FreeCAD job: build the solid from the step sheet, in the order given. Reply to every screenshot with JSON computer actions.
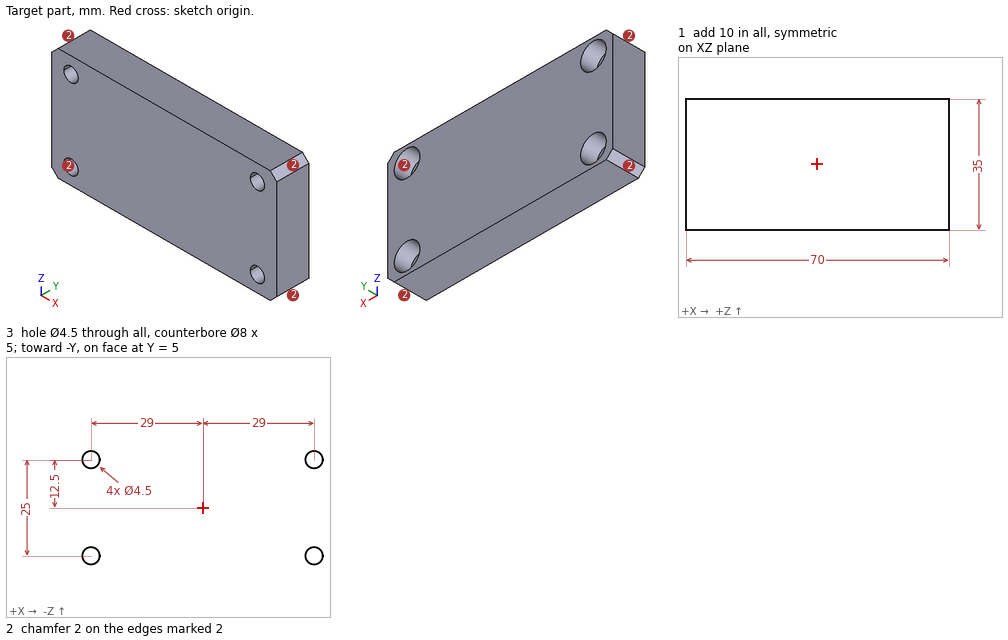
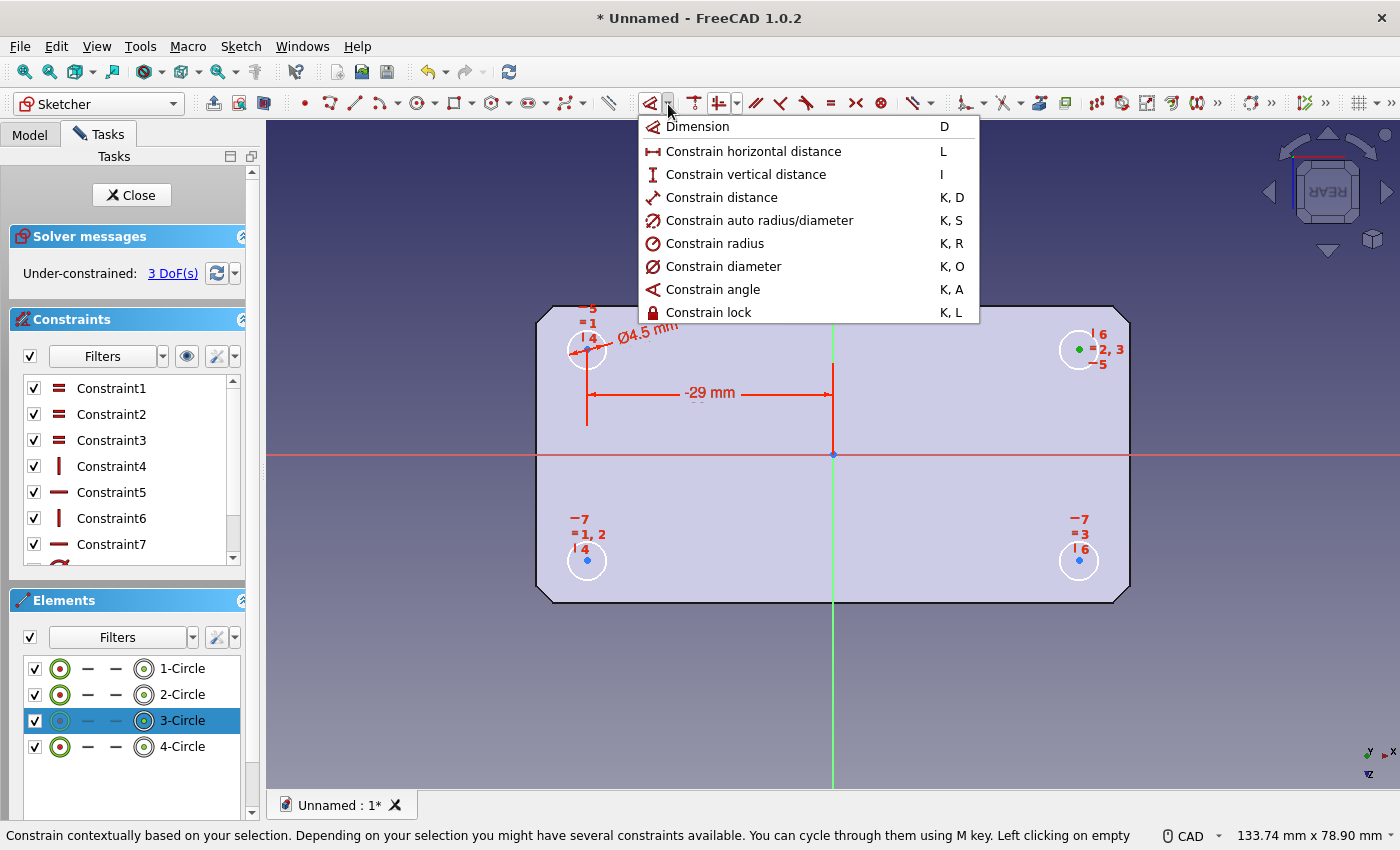
{"action": "left_click", "coordinate": [809, 152]}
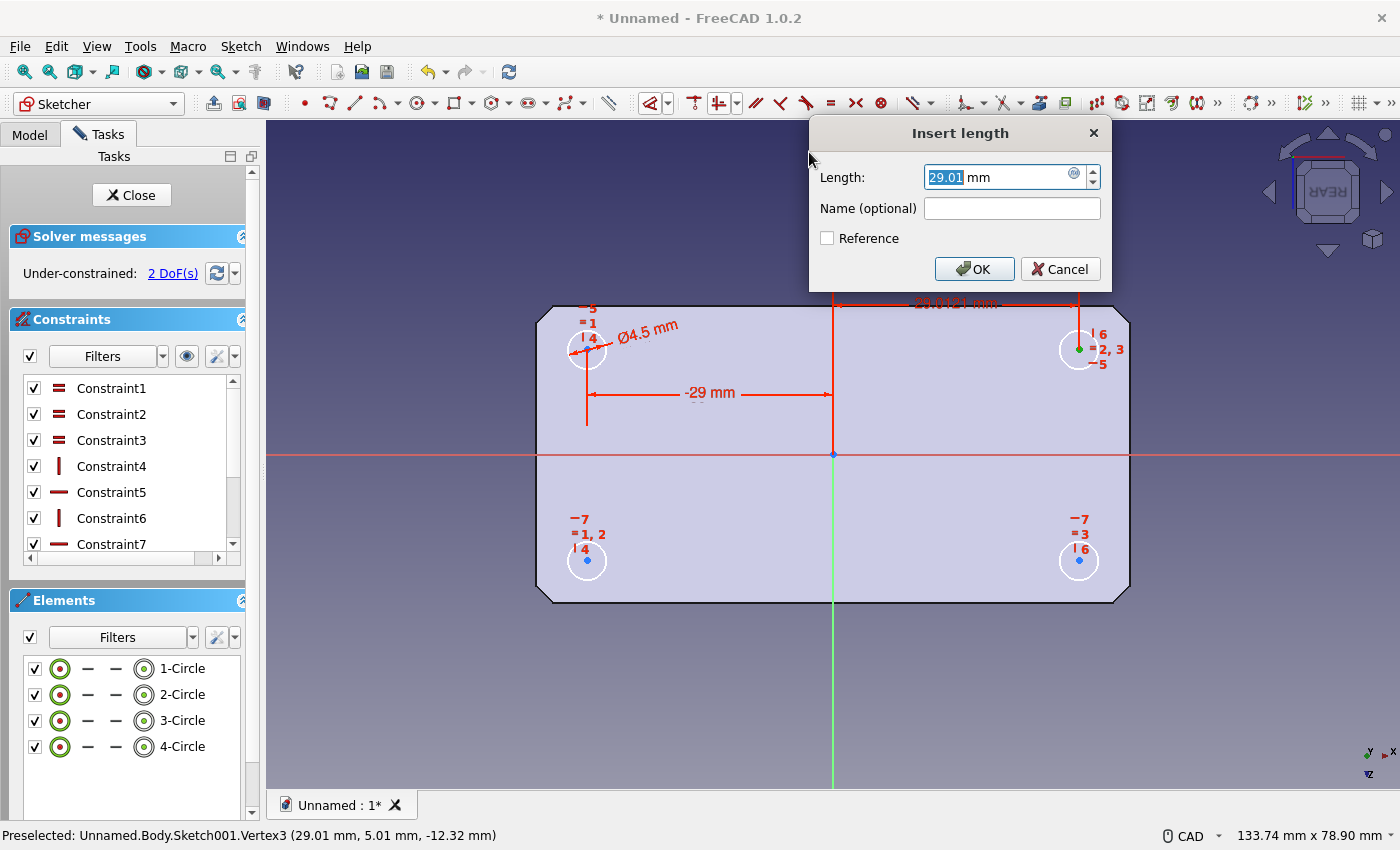
{"action": "type", "text": "29"}
{"action": "key", "text": "Return"}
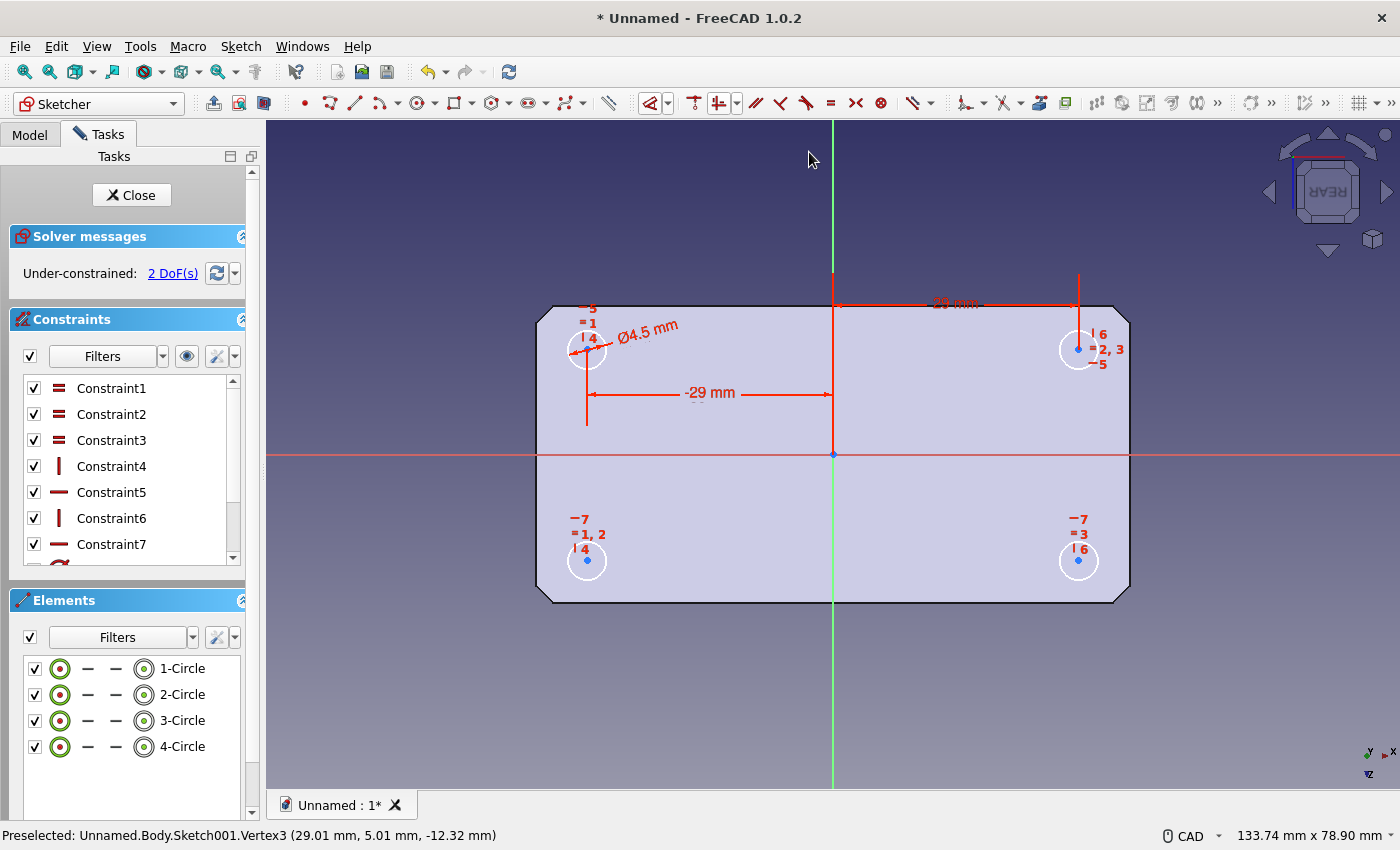
{"action": "left_click", "coordinate": [587, 350]}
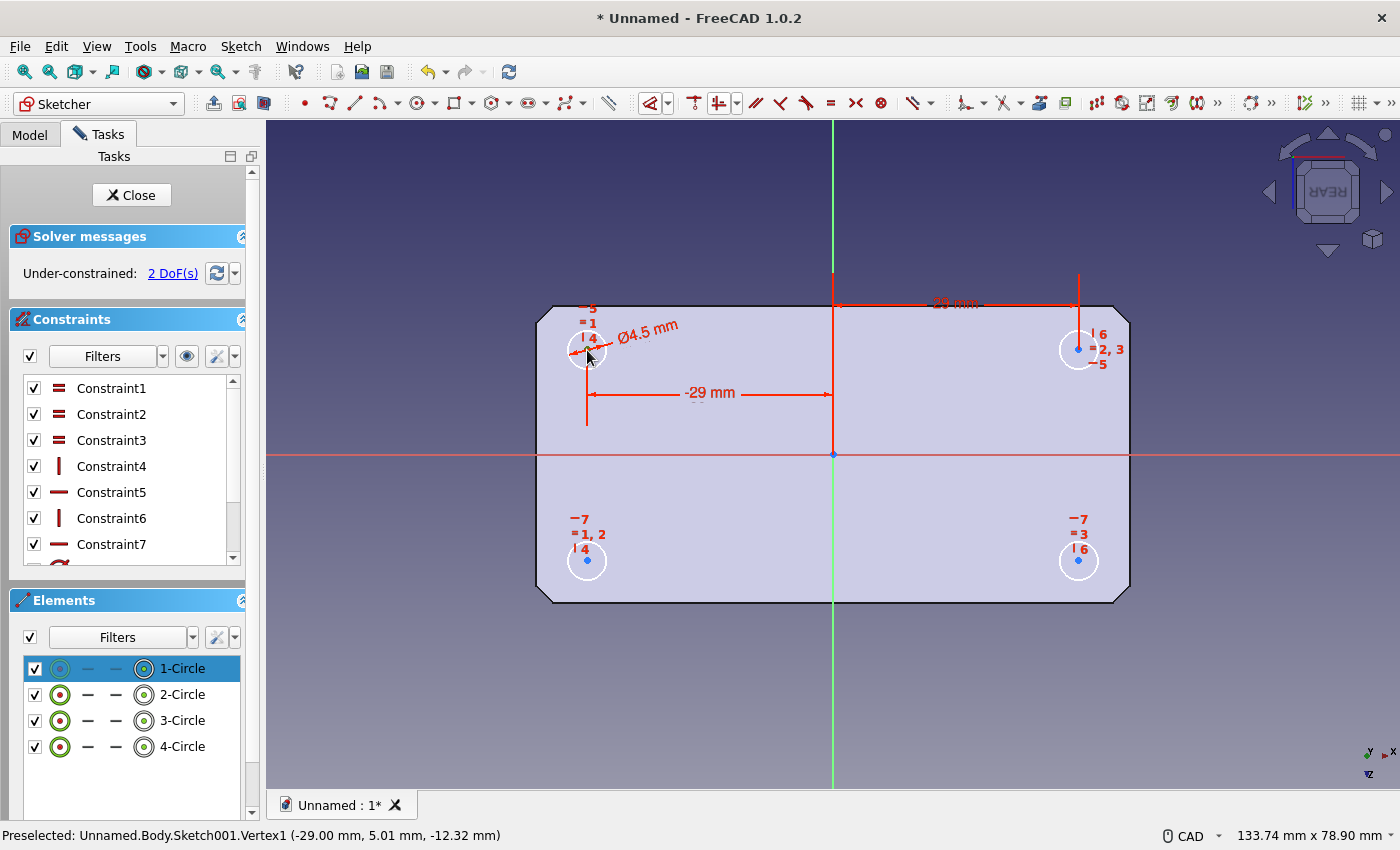
{"action": "left_click", "coordinate": [587, 561]}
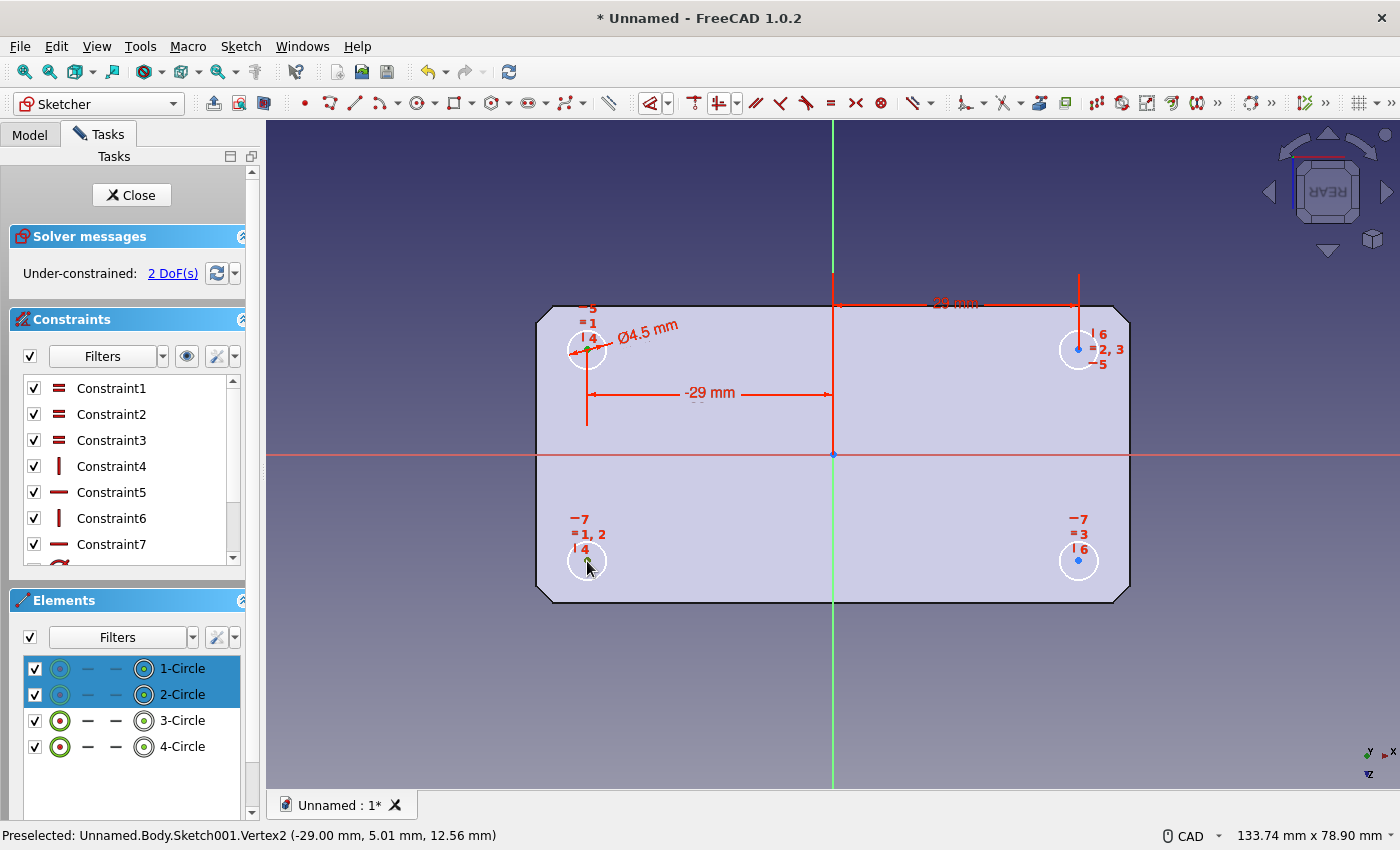
{"action": "key", "text": "i"}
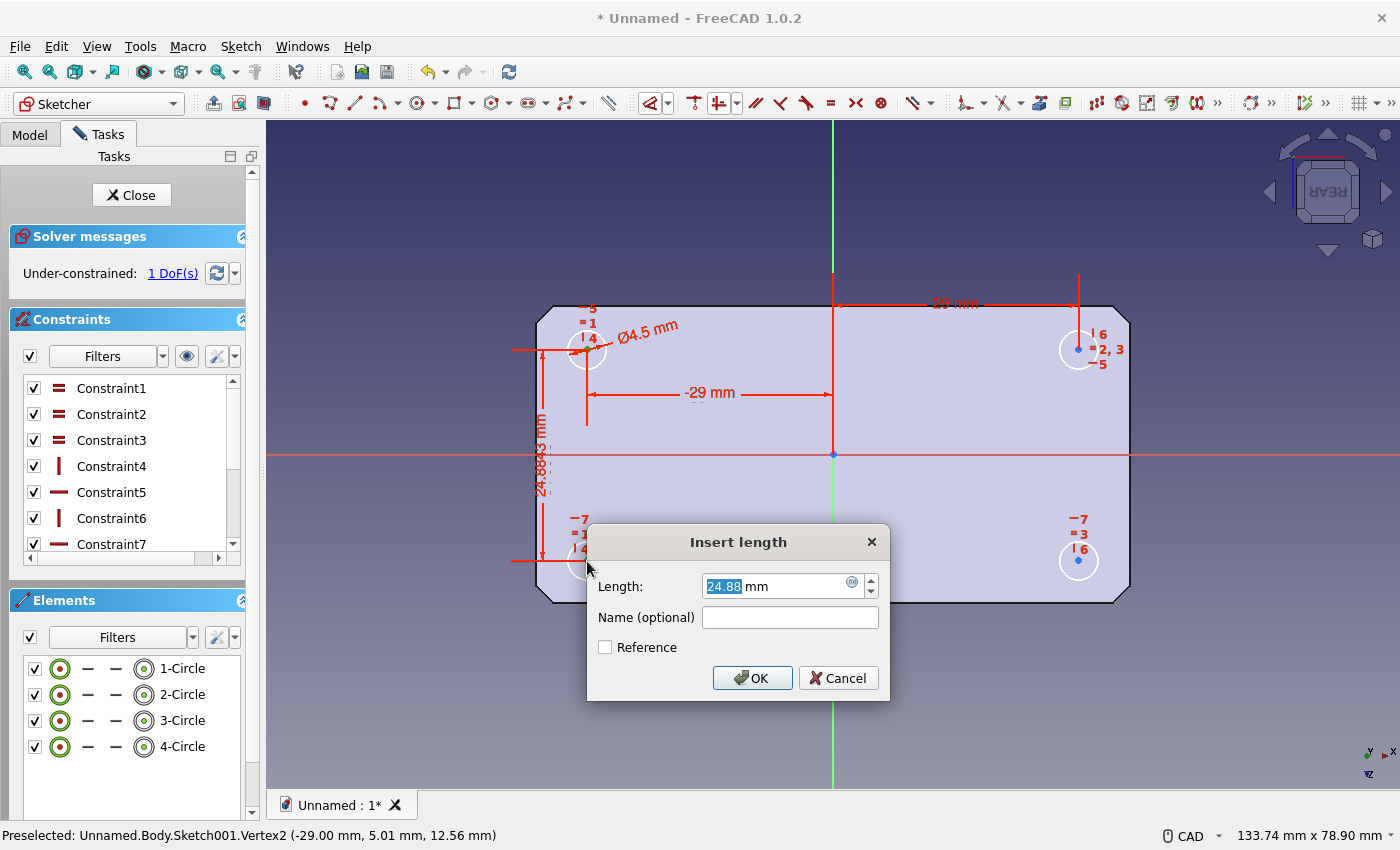
{"action": "type", "text": "25"}
{"action": "key", "text": "Return"}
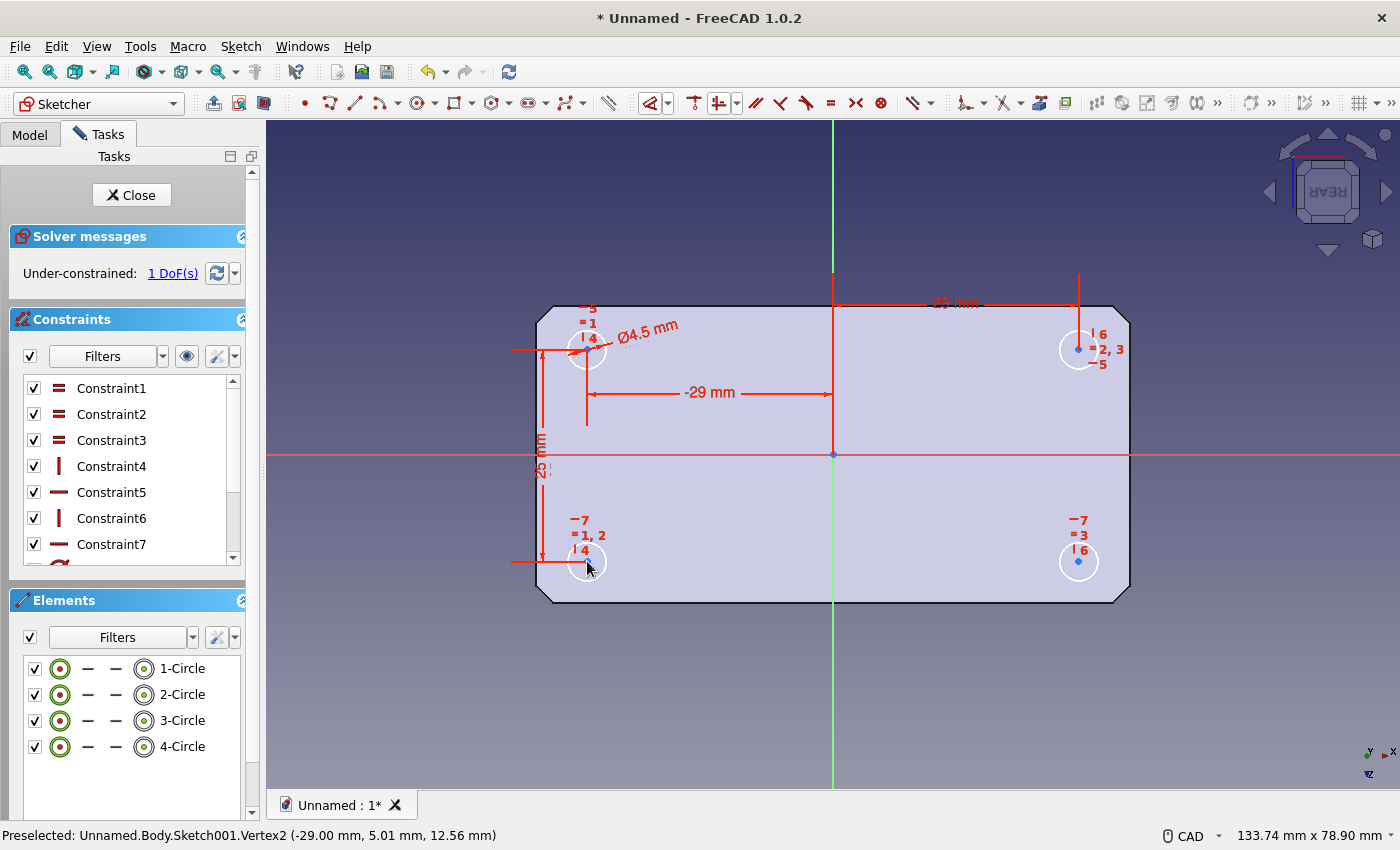
{"action": "left_click", "coordinate": [587, 350]}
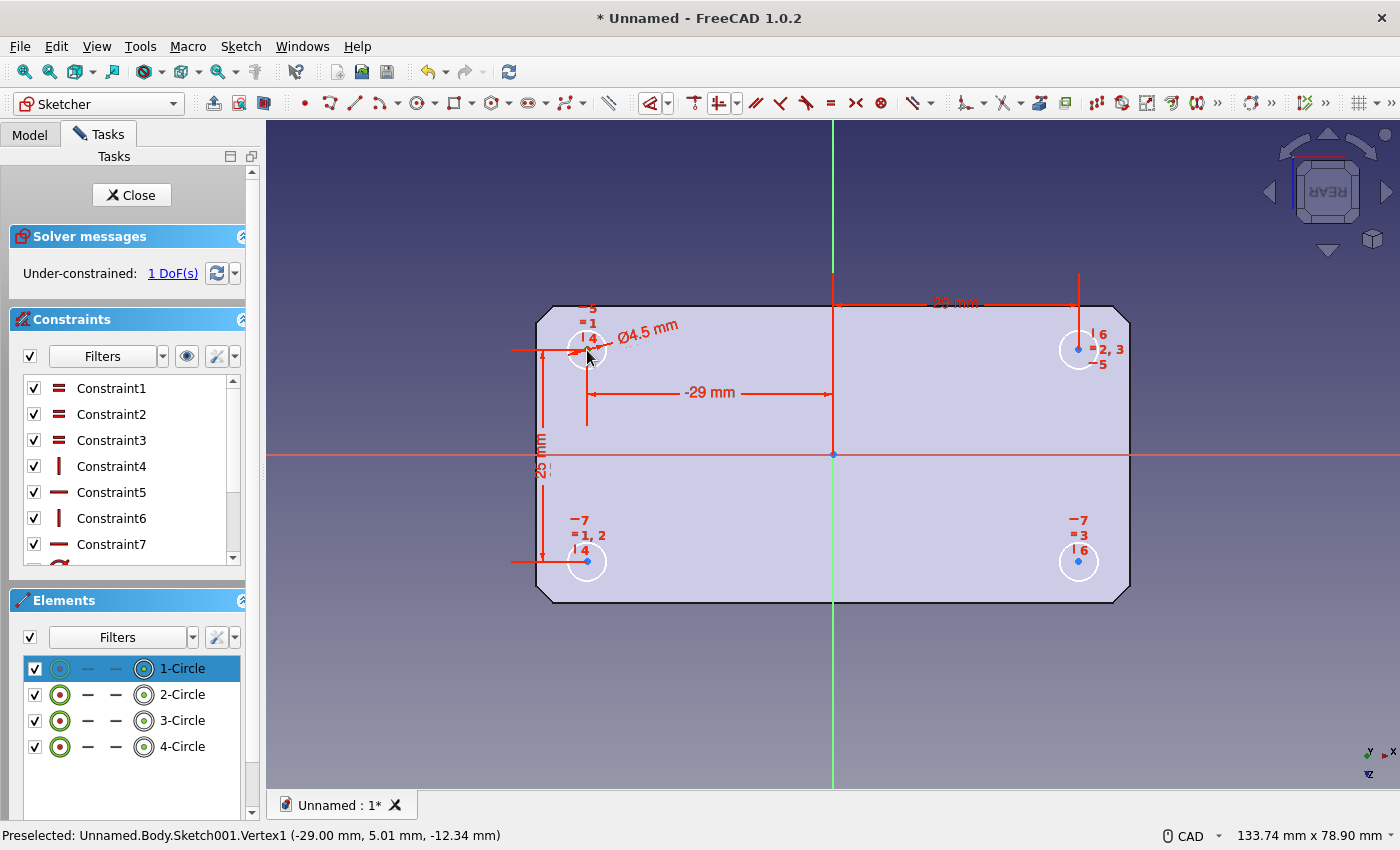
{"action": "key", "text": "i"}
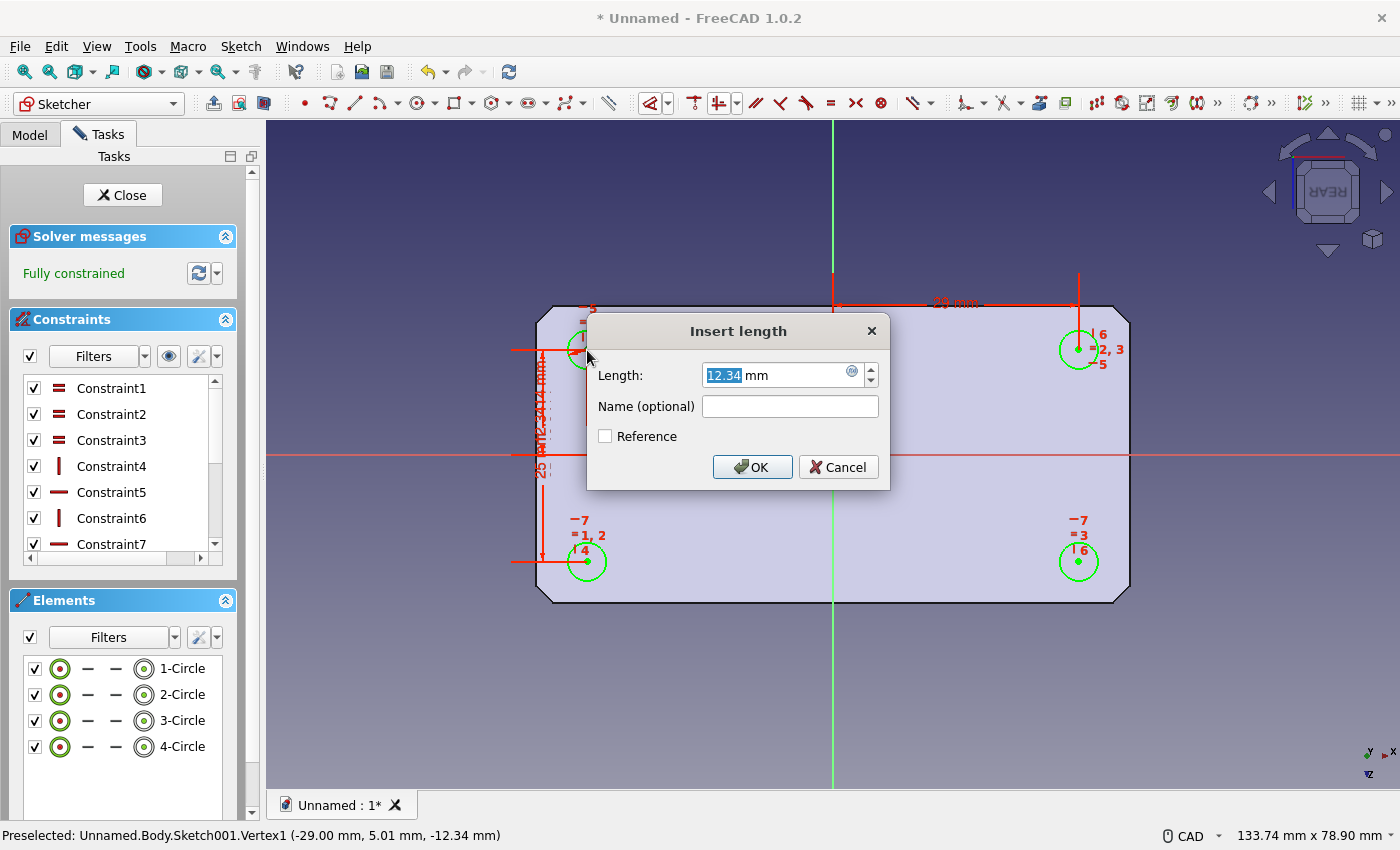
{"action": "type", "text": "12.5"}
{"action": "key", "text": "Return"}